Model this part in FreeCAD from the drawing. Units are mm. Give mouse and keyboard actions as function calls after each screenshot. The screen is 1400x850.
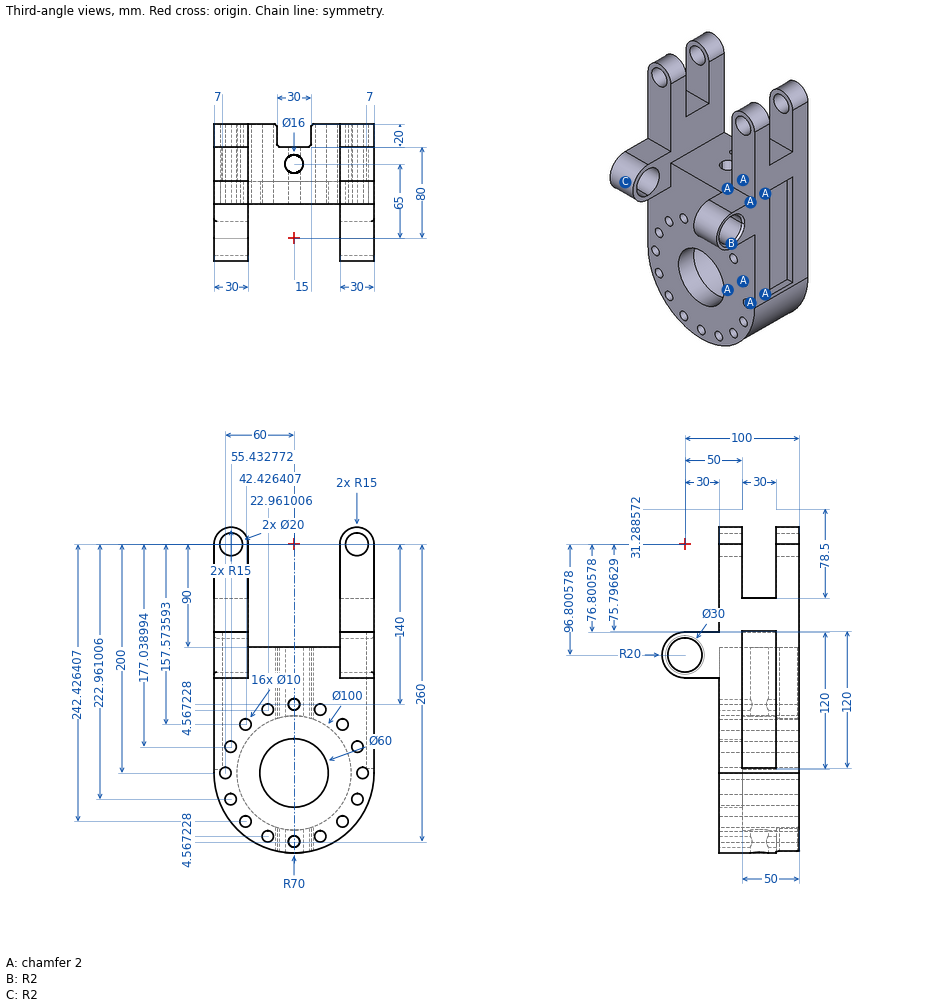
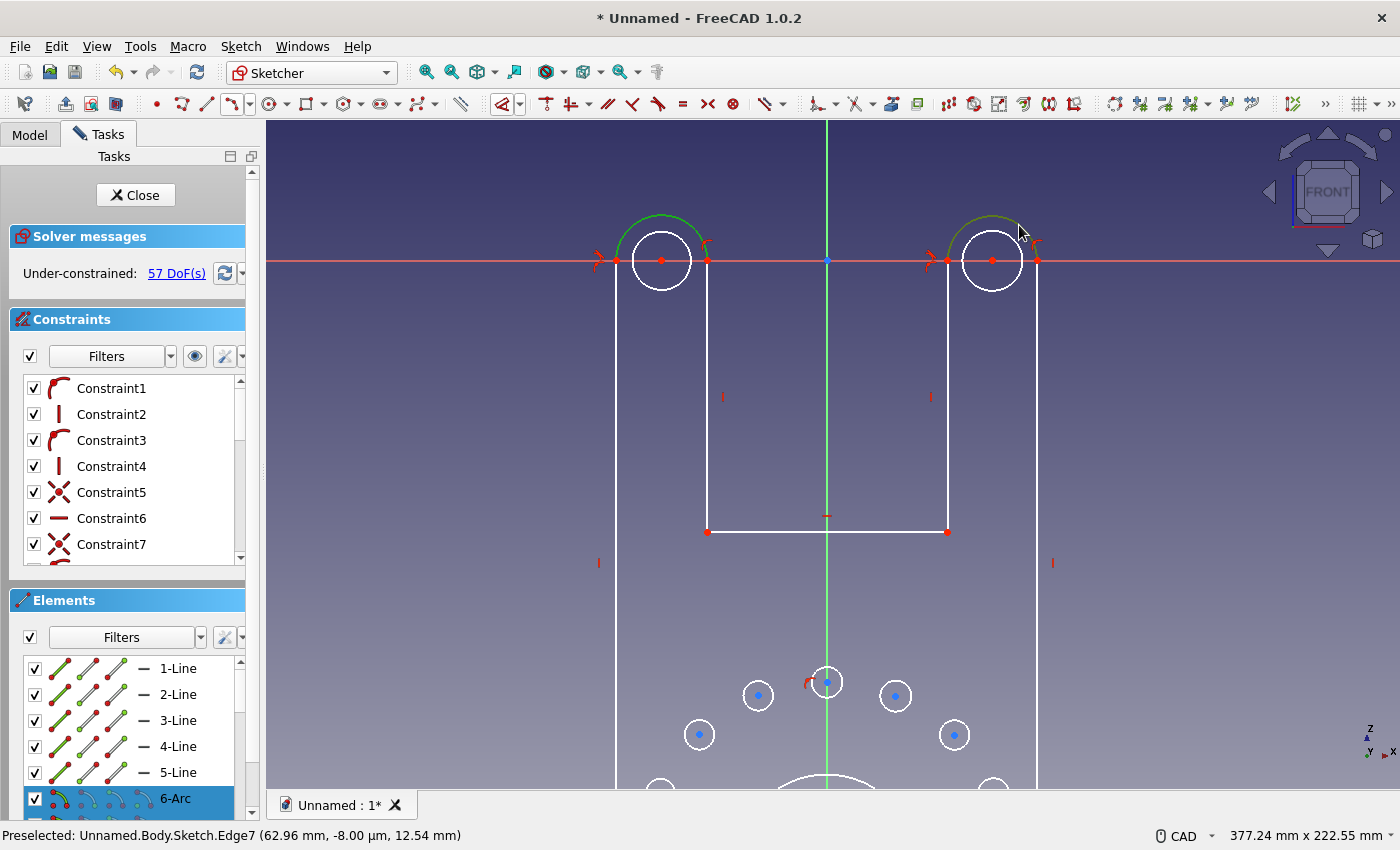
key(e)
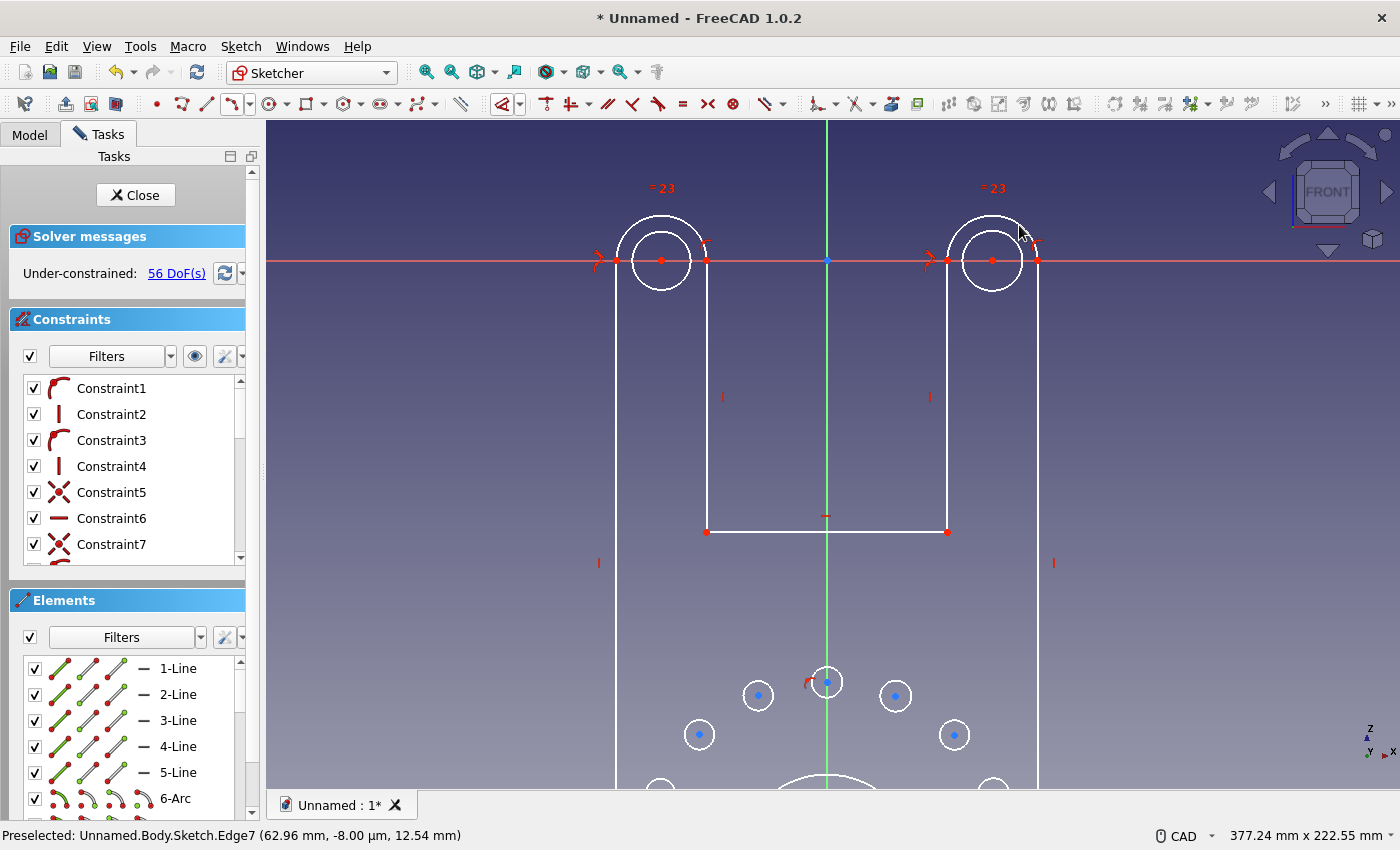
click(682, 240)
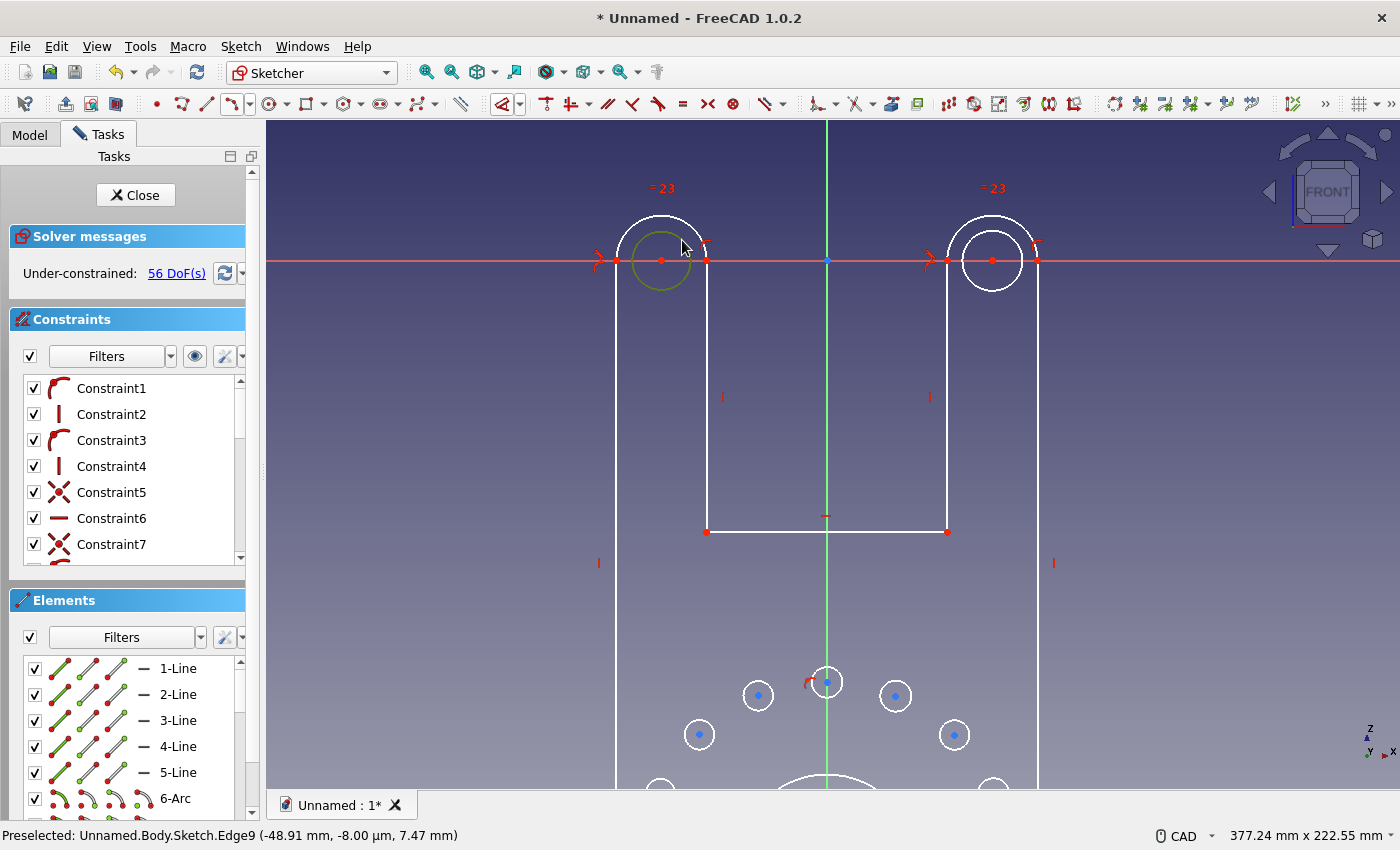
click(1014, 240)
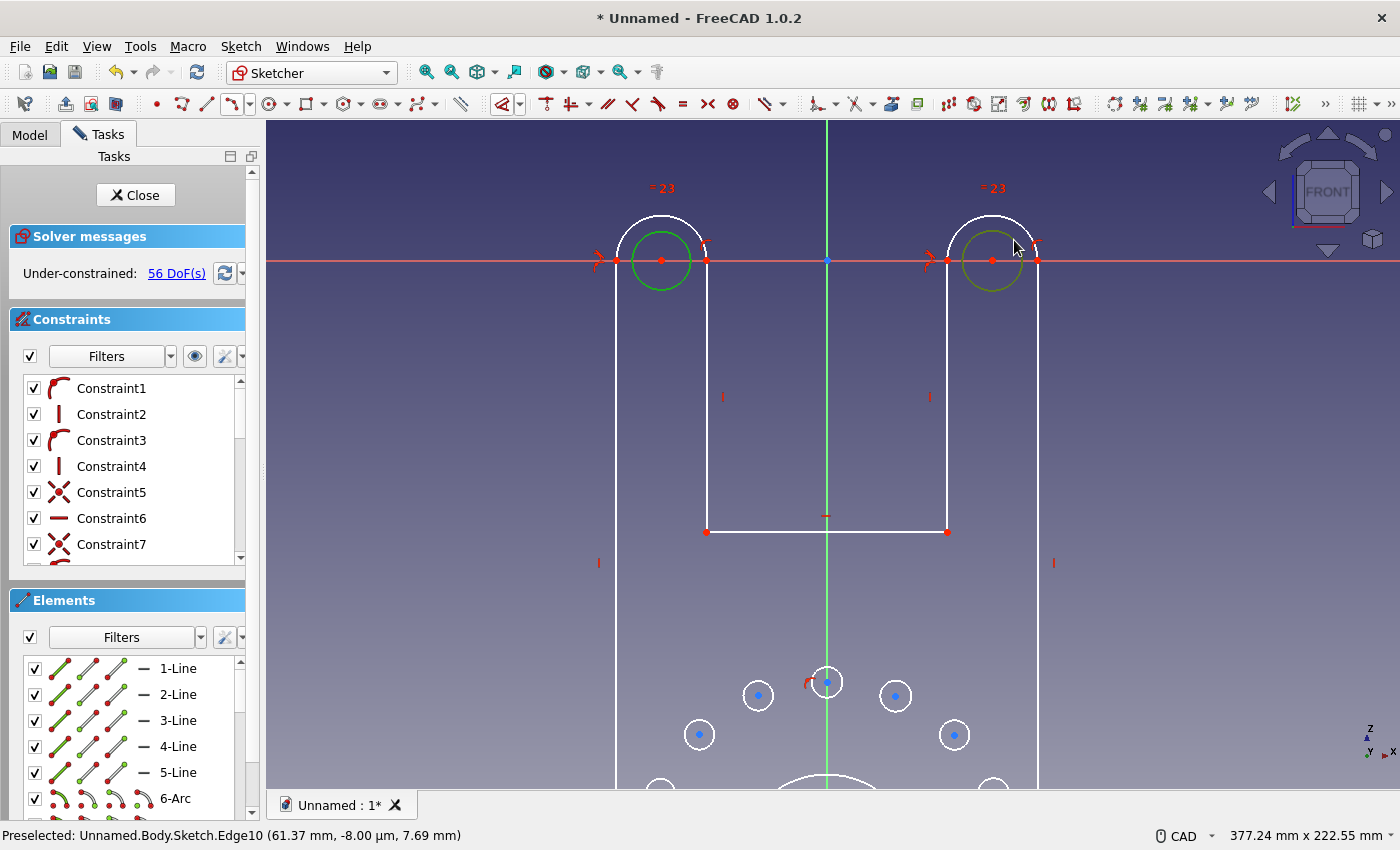
key(e)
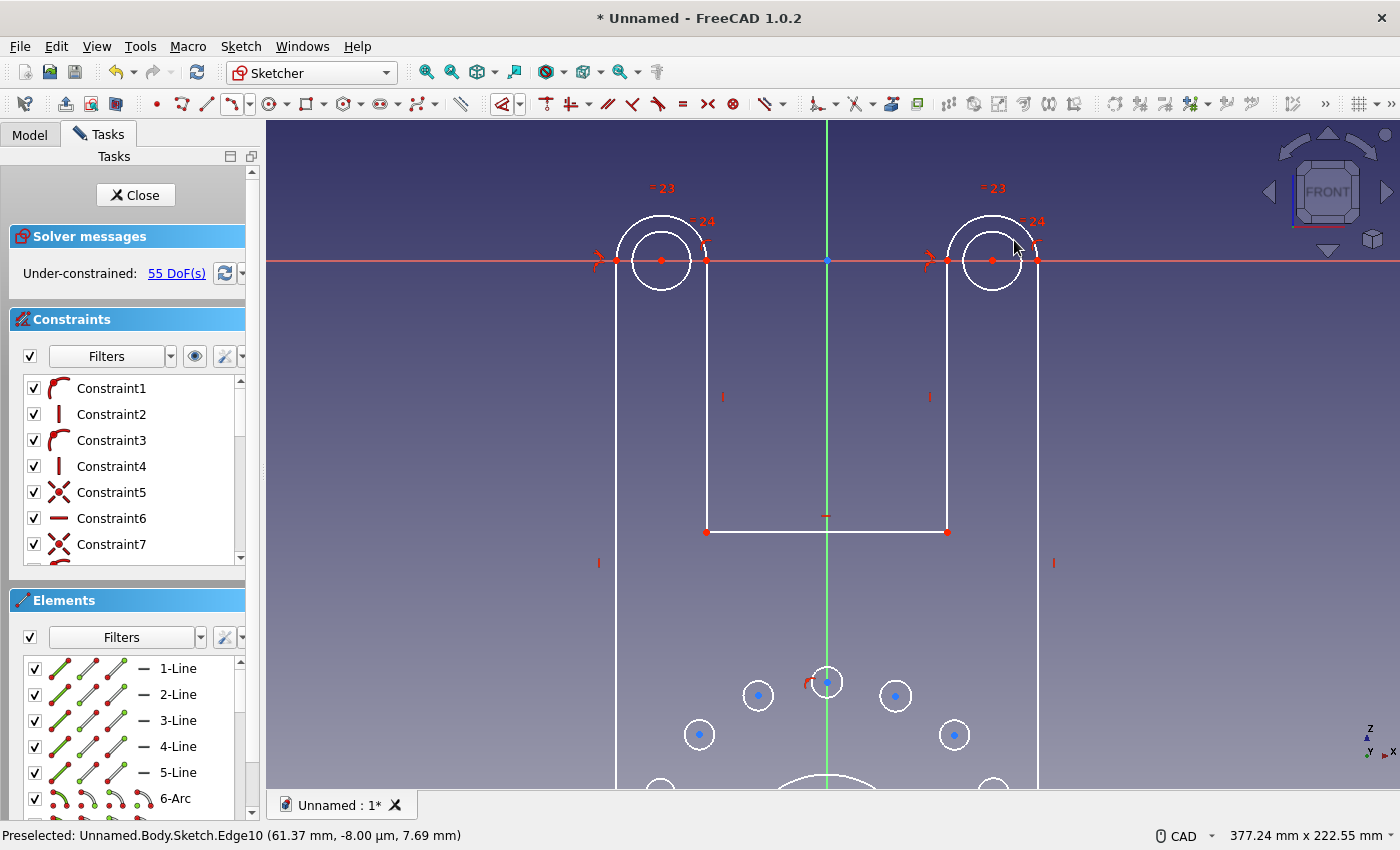
click(710, 724)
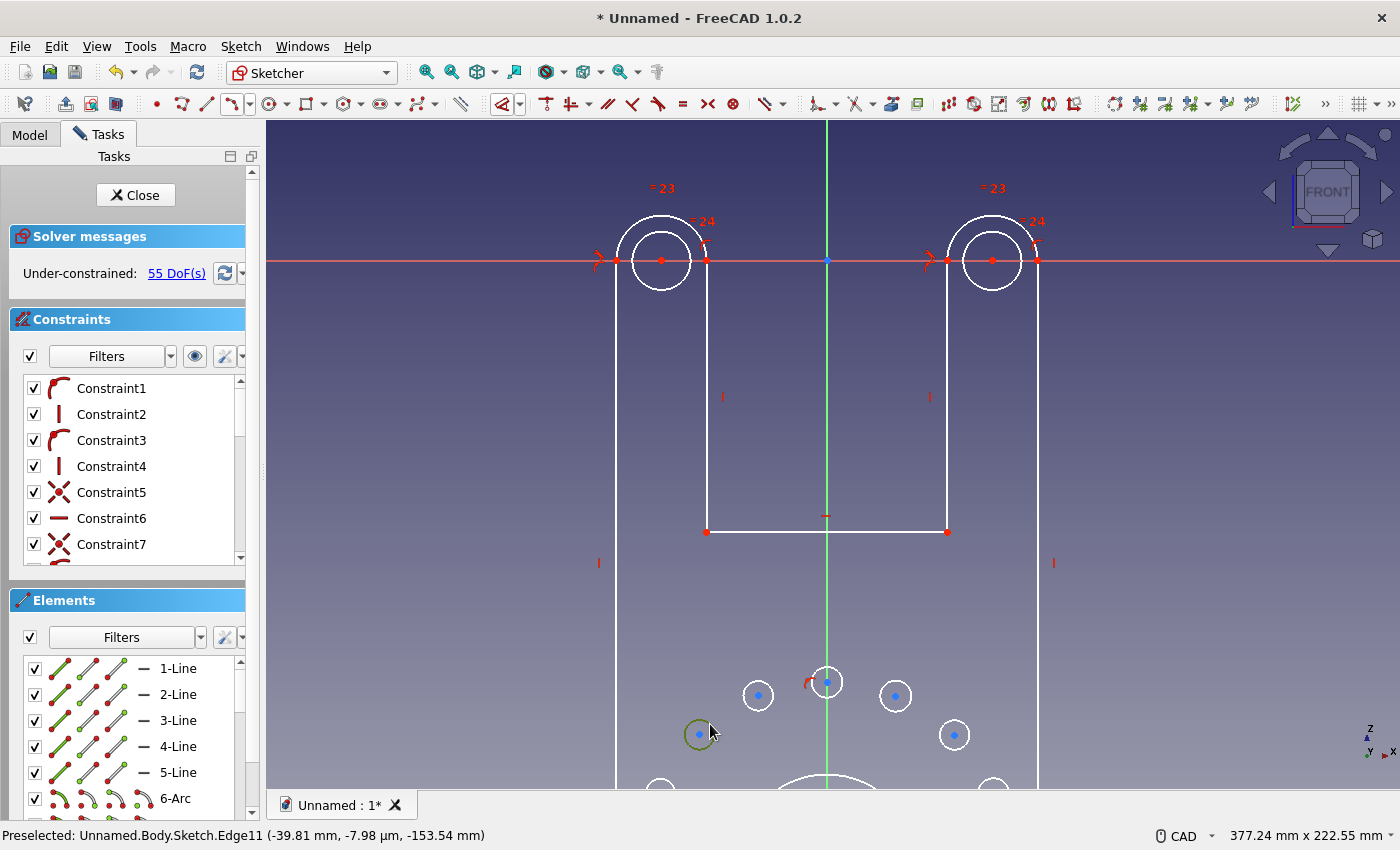
scroll(688, 224, down, 3)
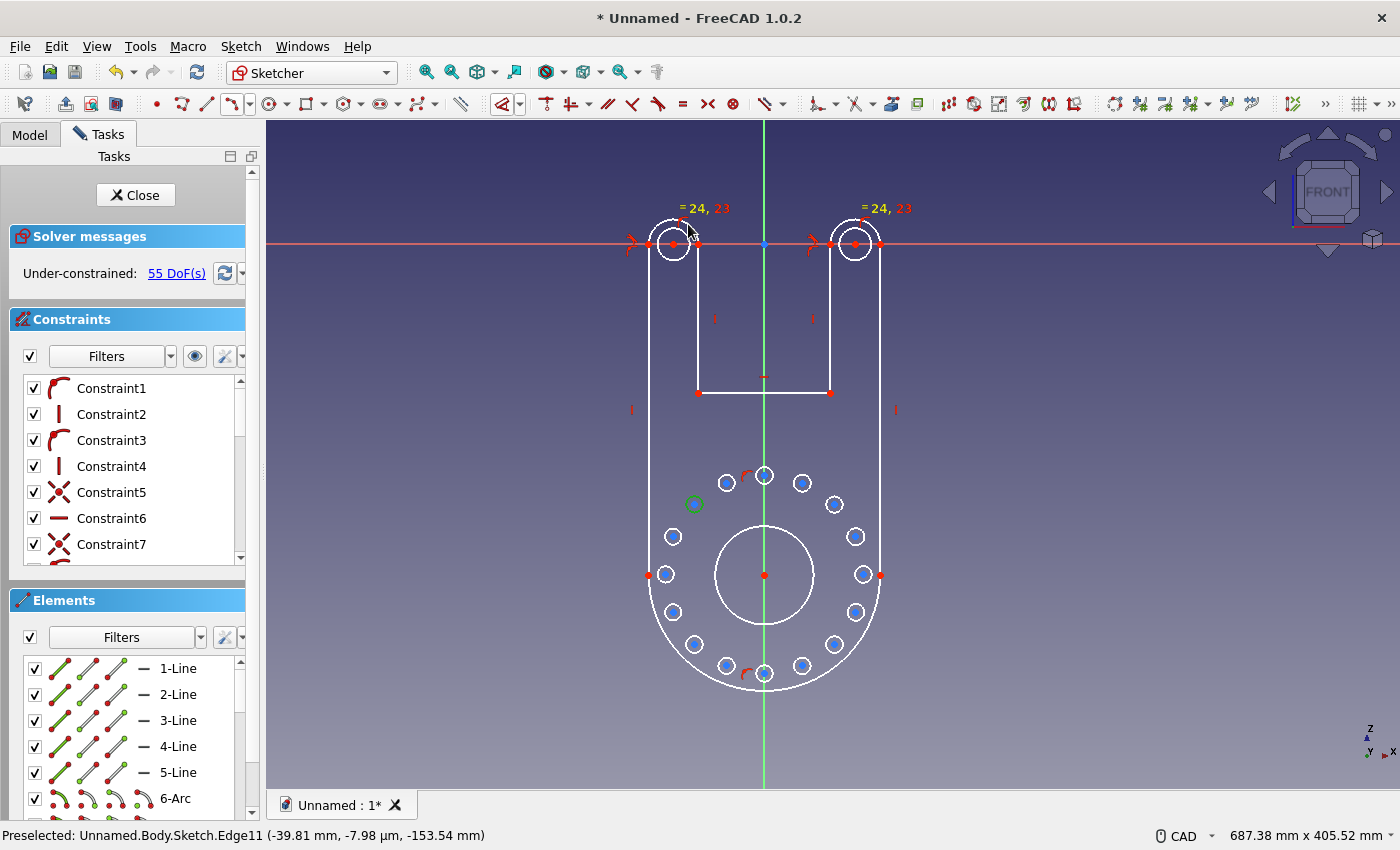
scroll(679, 531, up, 3)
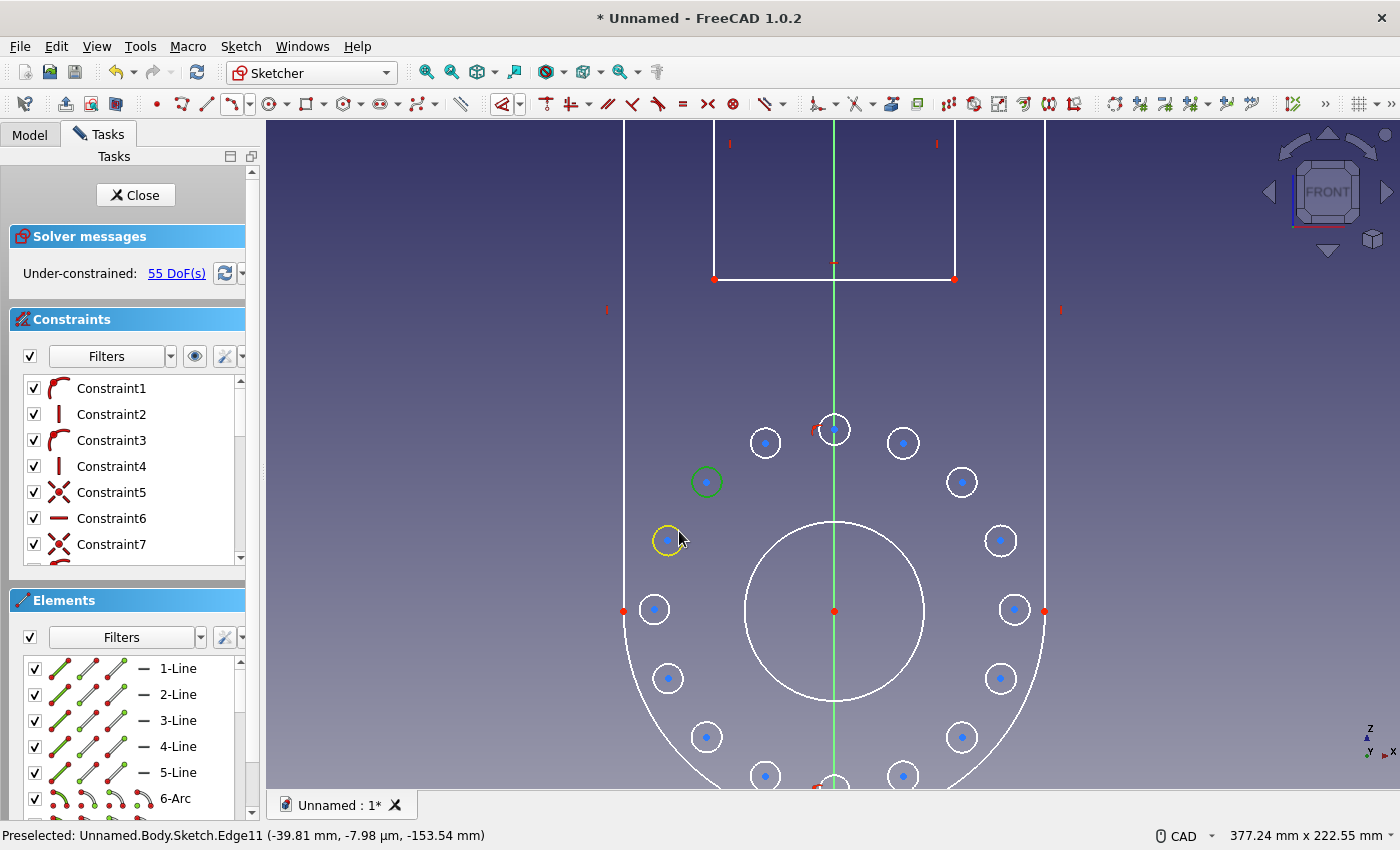
click(678, 530)